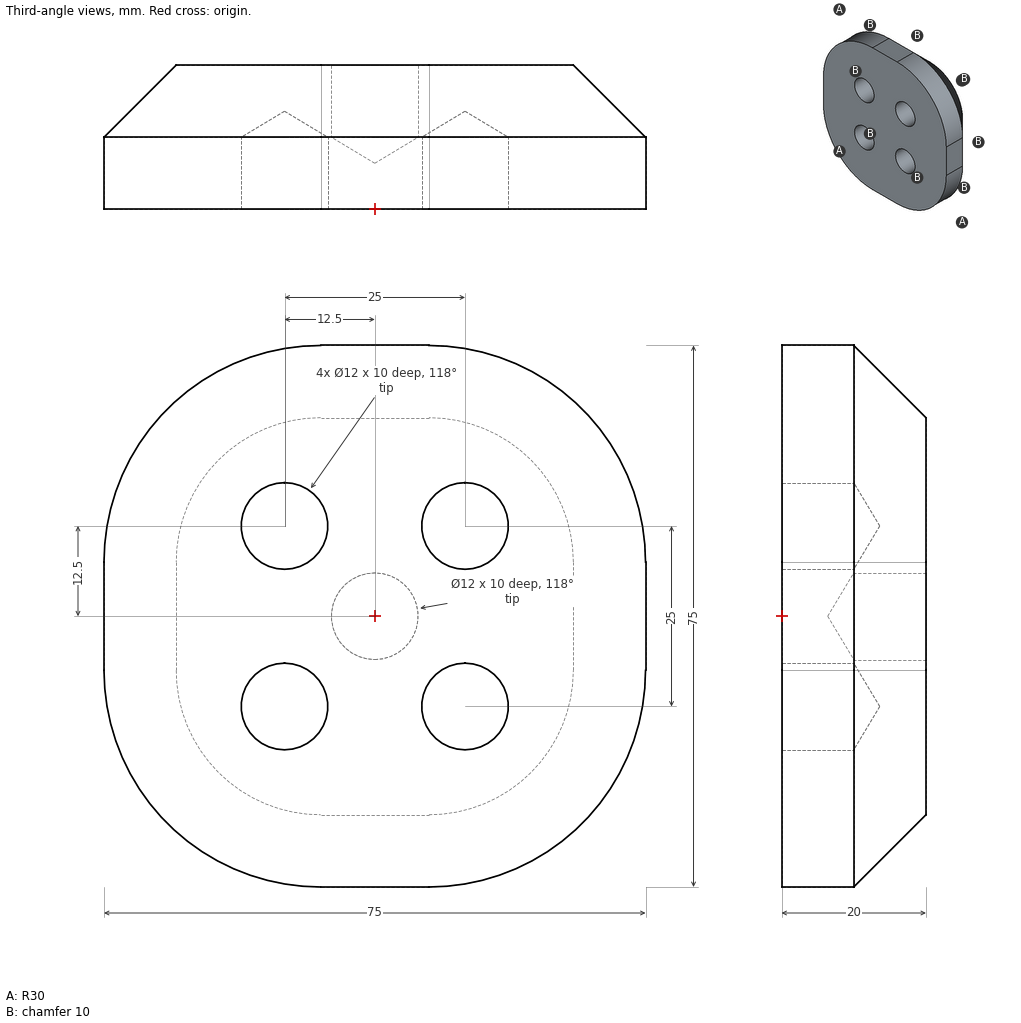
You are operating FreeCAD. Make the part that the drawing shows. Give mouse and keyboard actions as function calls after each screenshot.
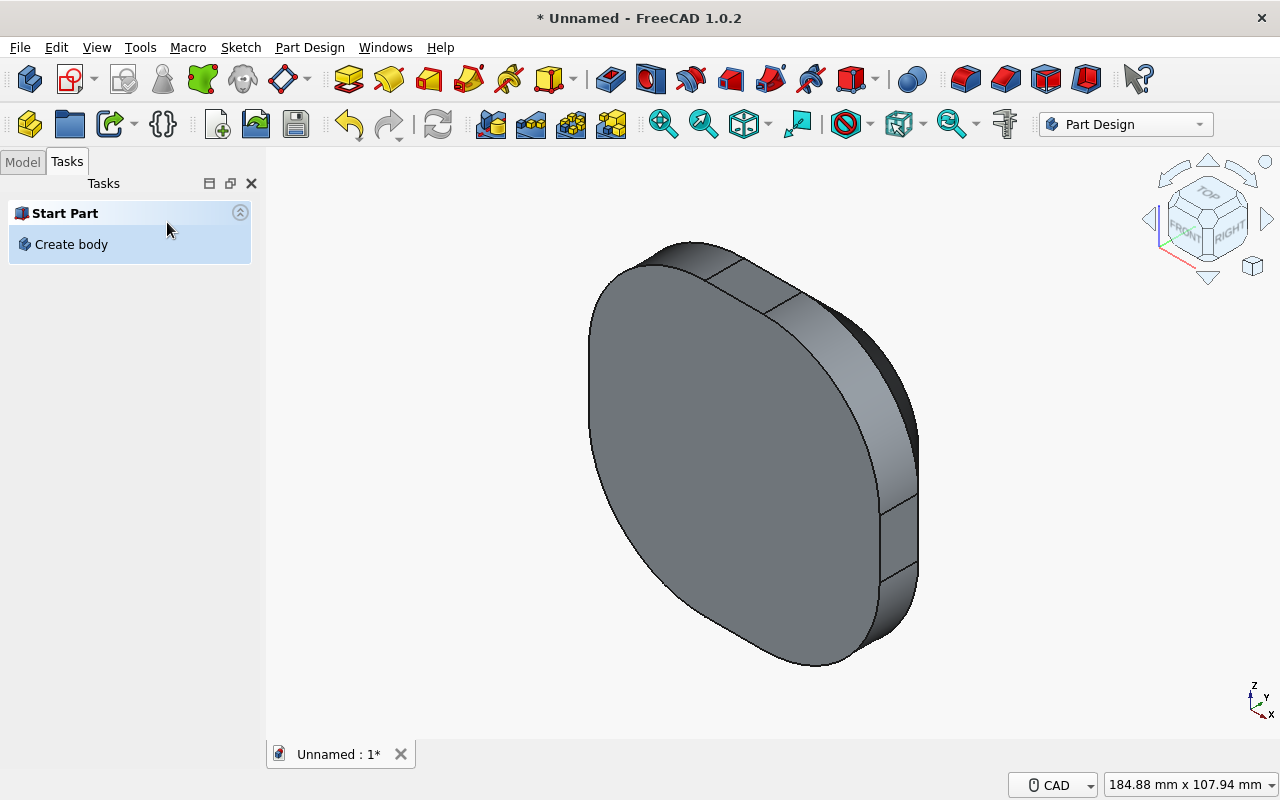
click(734, 464)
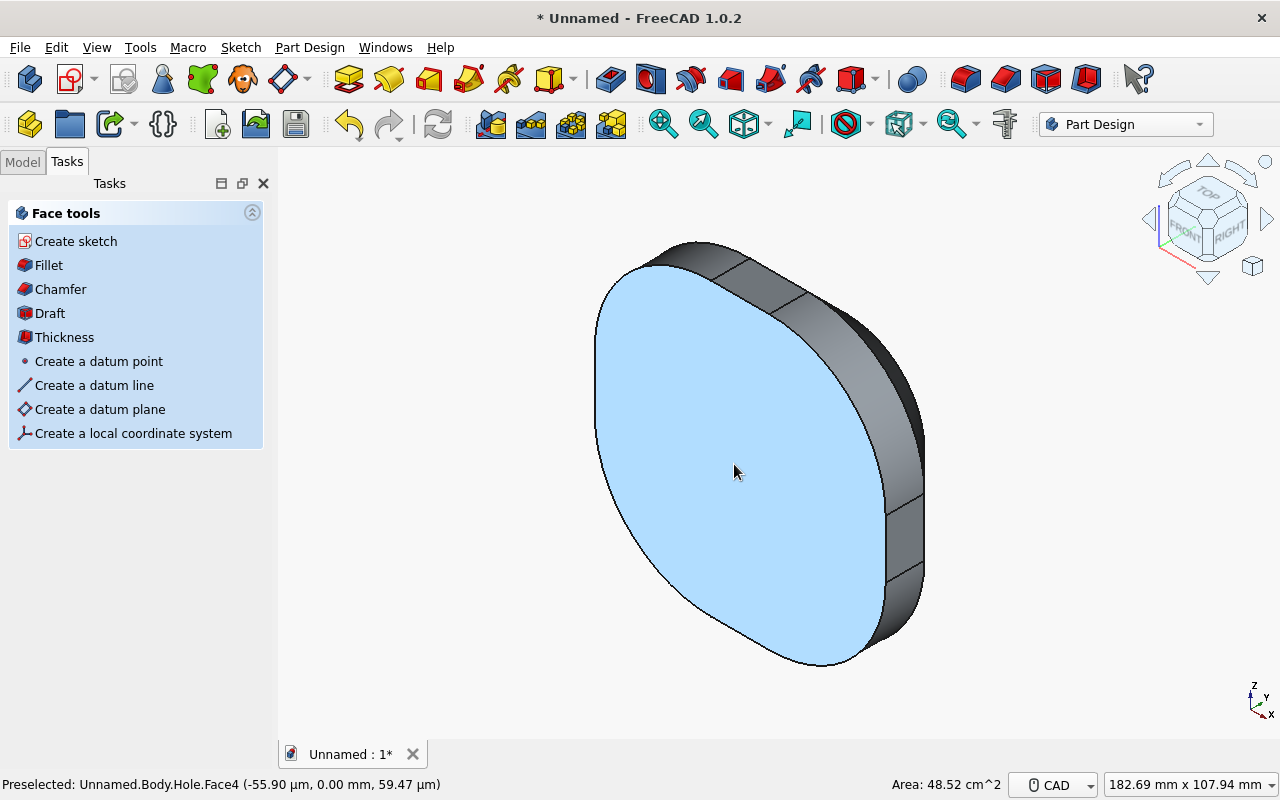
click(70, 80)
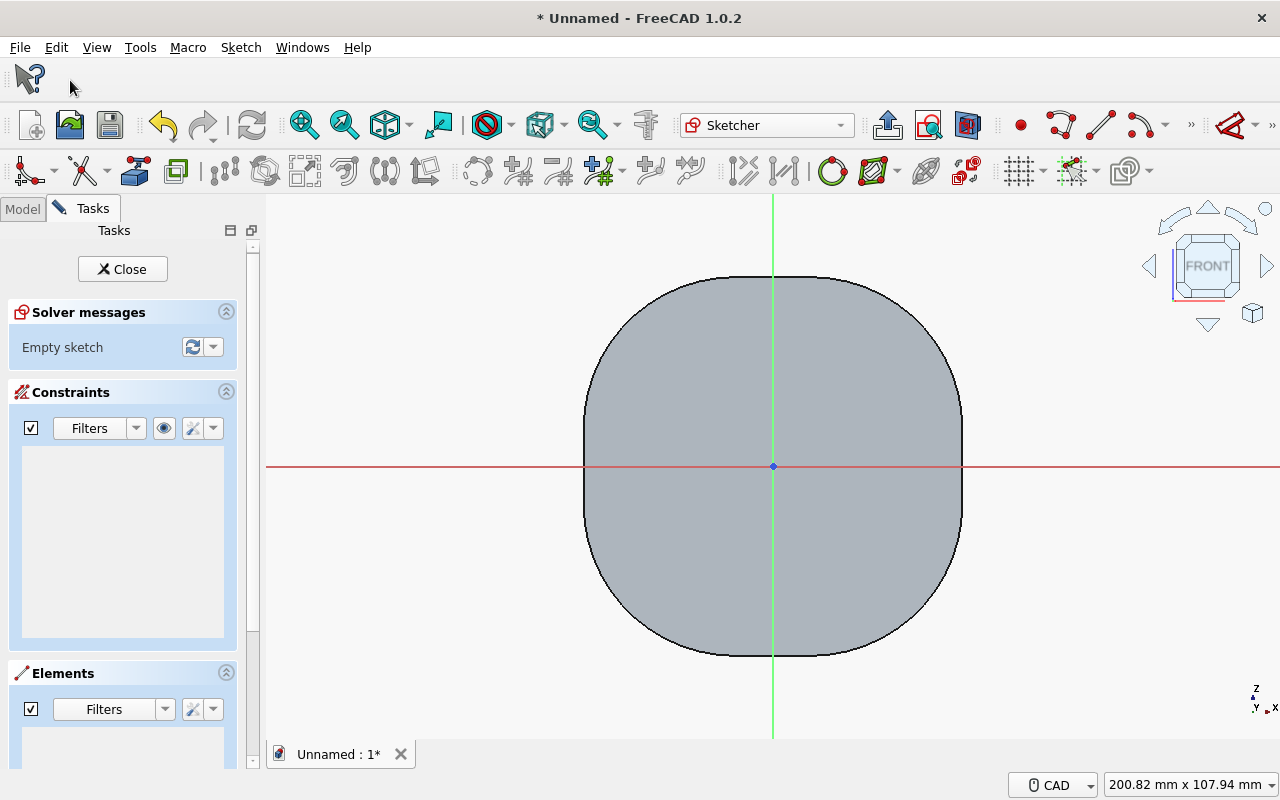
scroll(856, 467, up, 3)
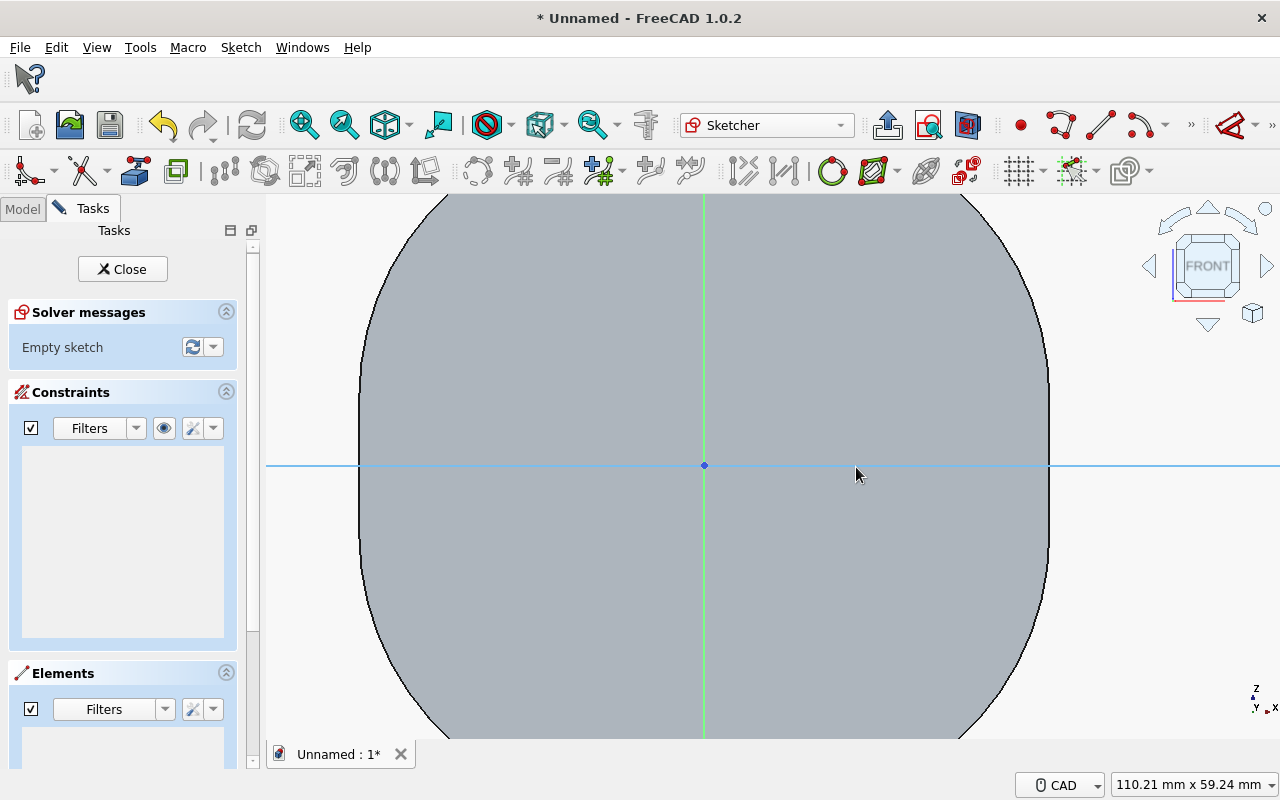
key(g)
key(c)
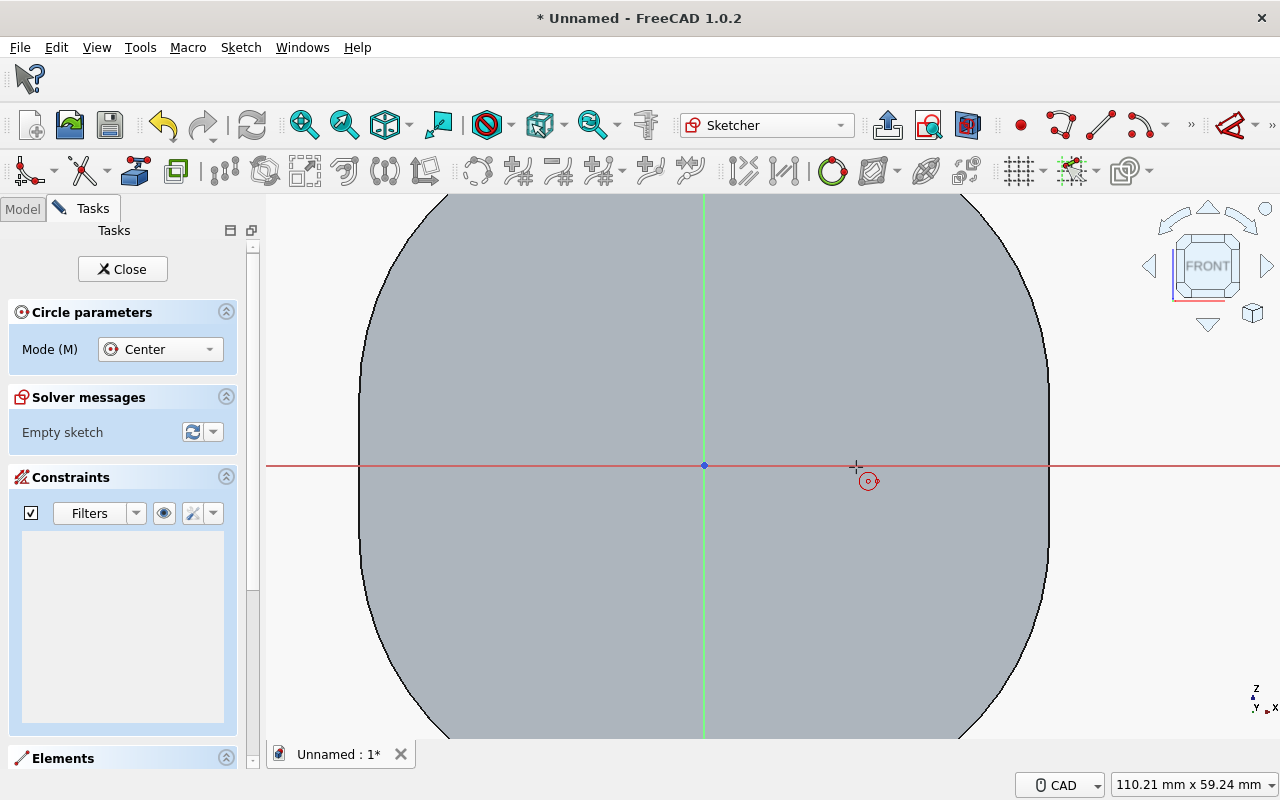
click(589, 351)
click(628, 312)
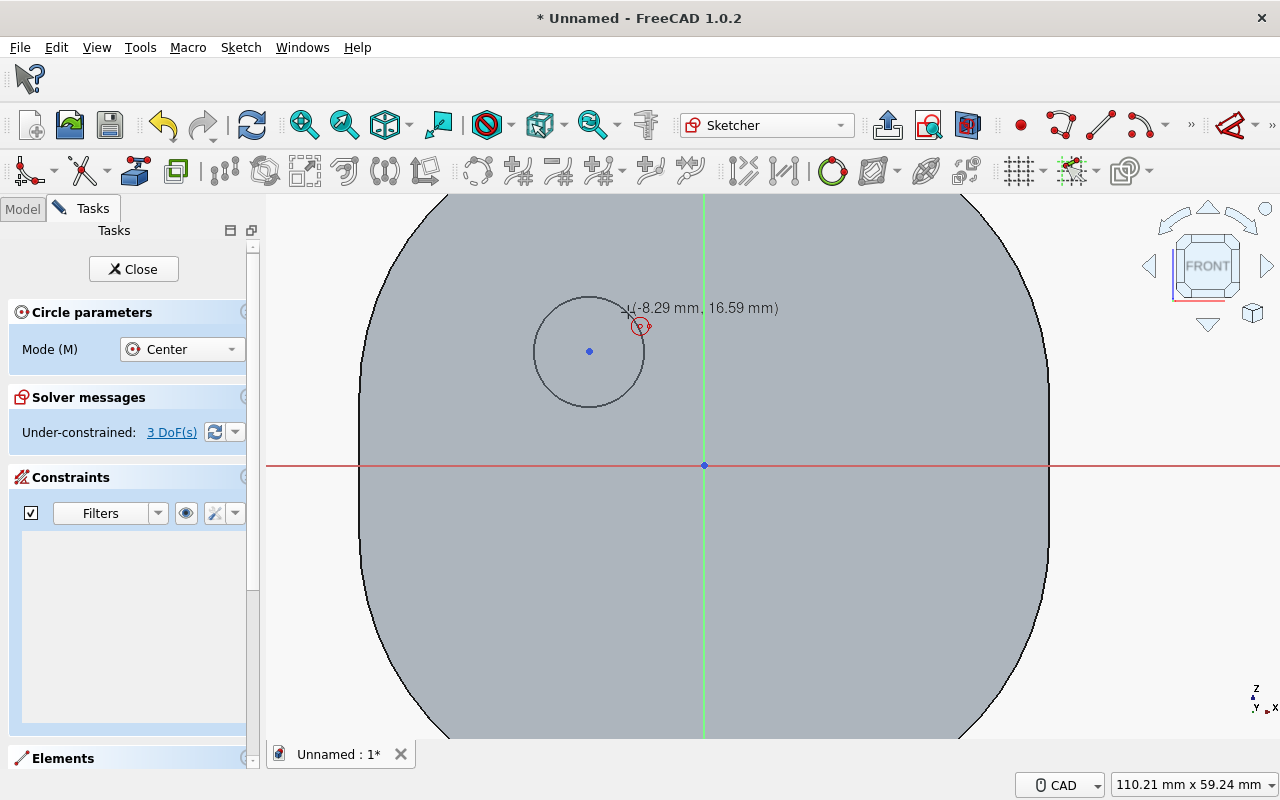
click(819, 351)
click(858, 312)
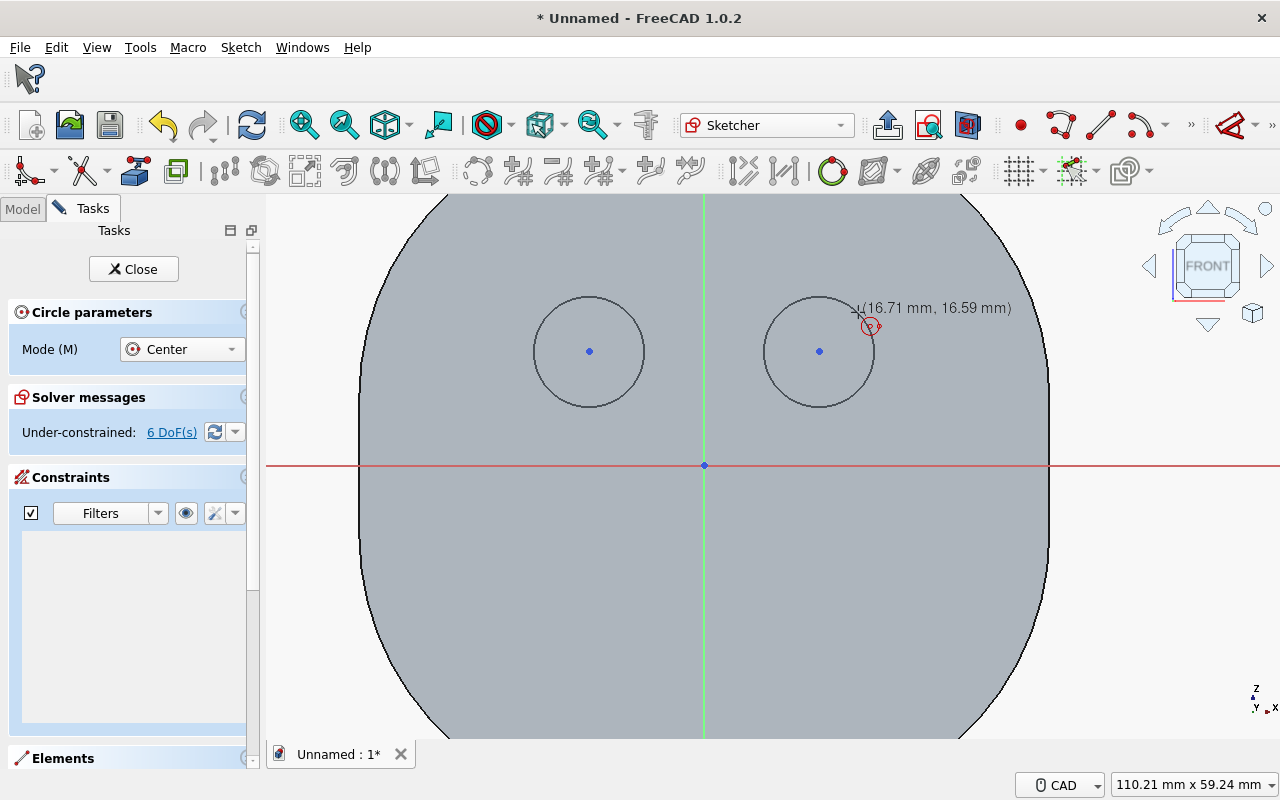
click(819, 581)
click(858, 542)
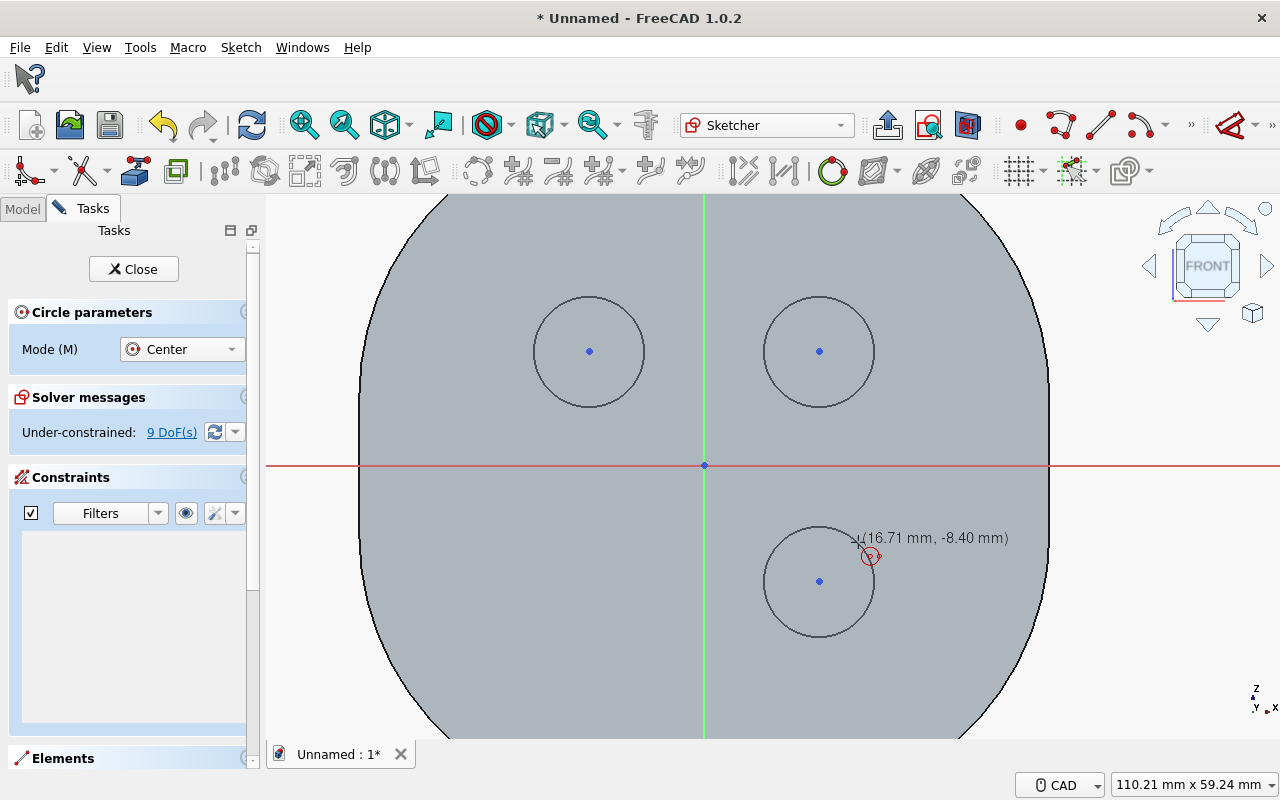
click(589, 581)
click(628, 542)
key(Escape)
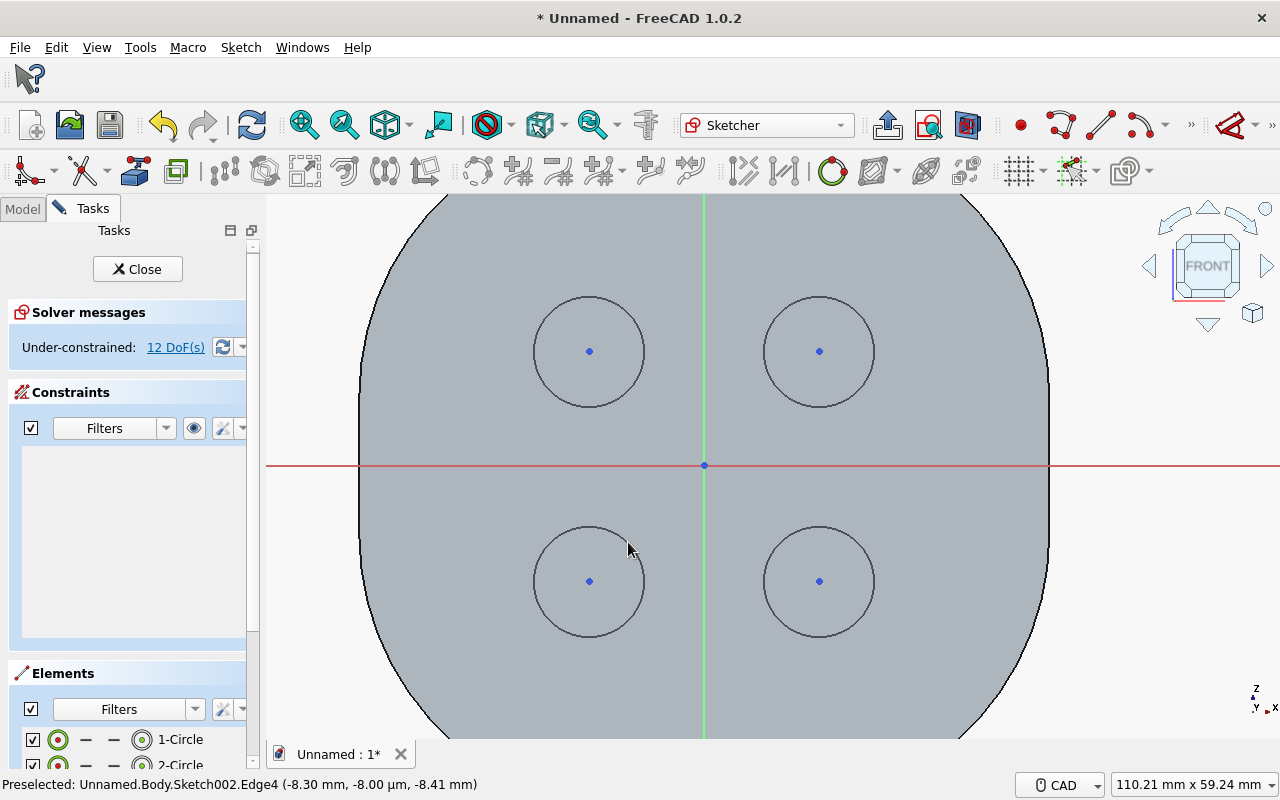
click(628, 313)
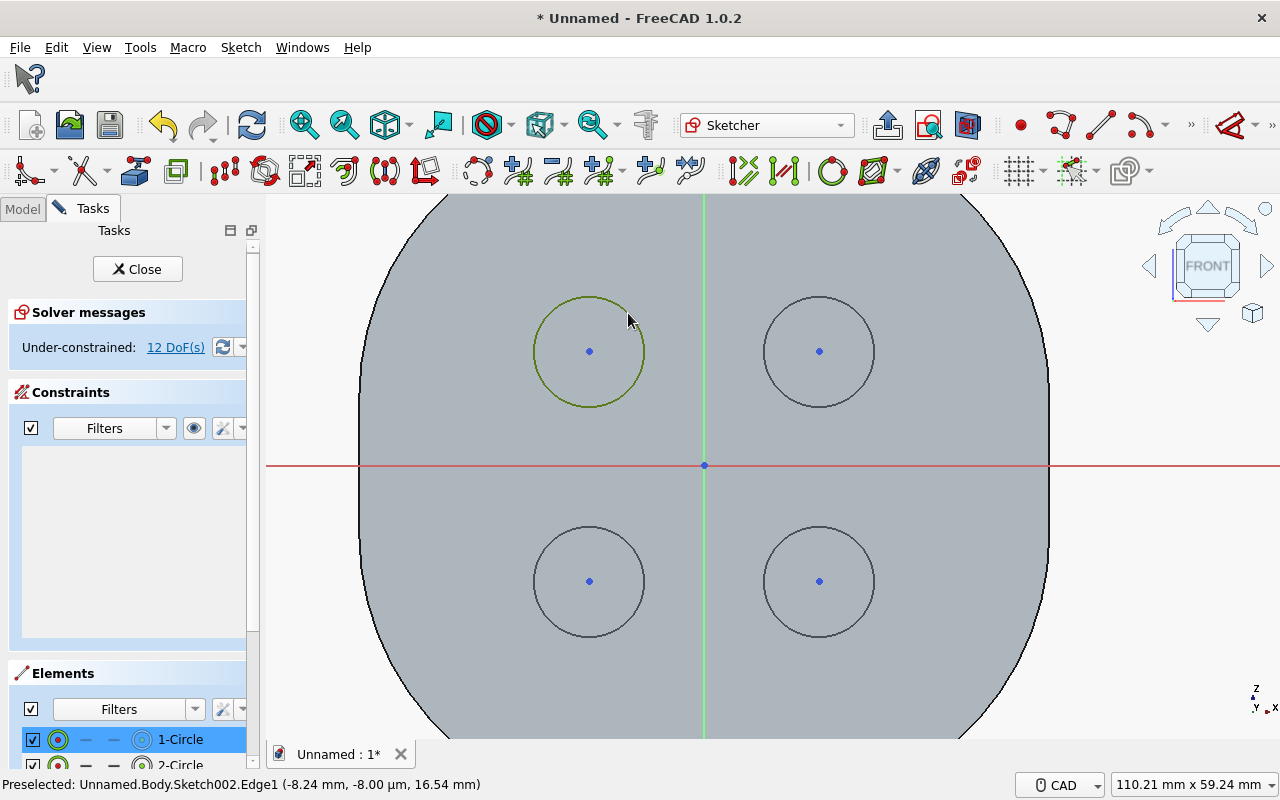
click(858, 313)